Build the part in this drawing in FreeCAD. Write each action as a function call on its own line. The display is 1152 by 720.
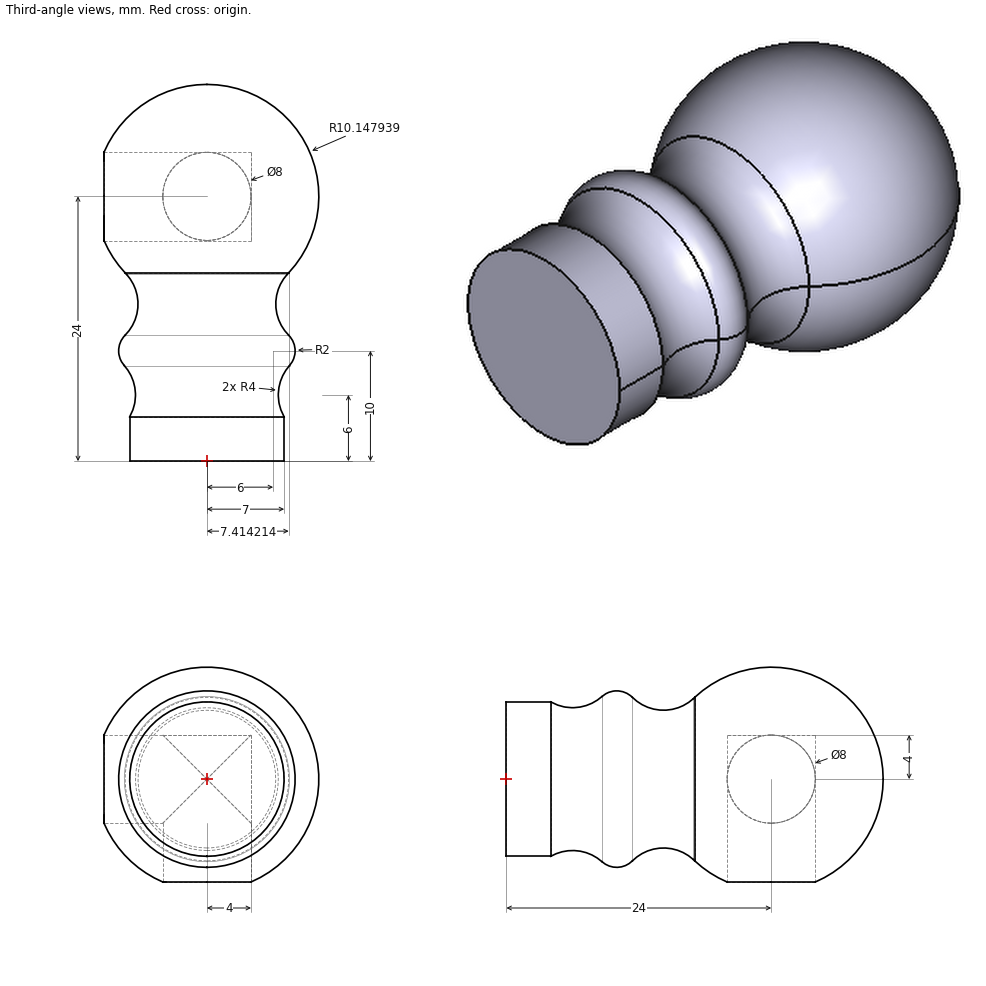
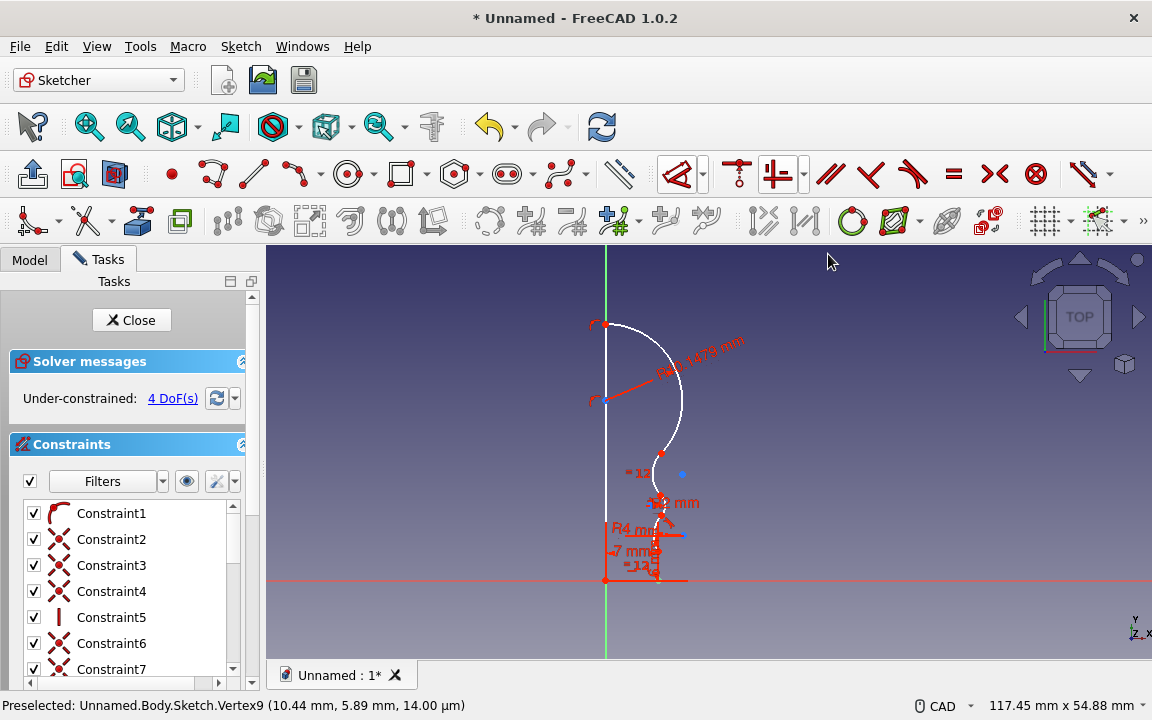
click(650, 506)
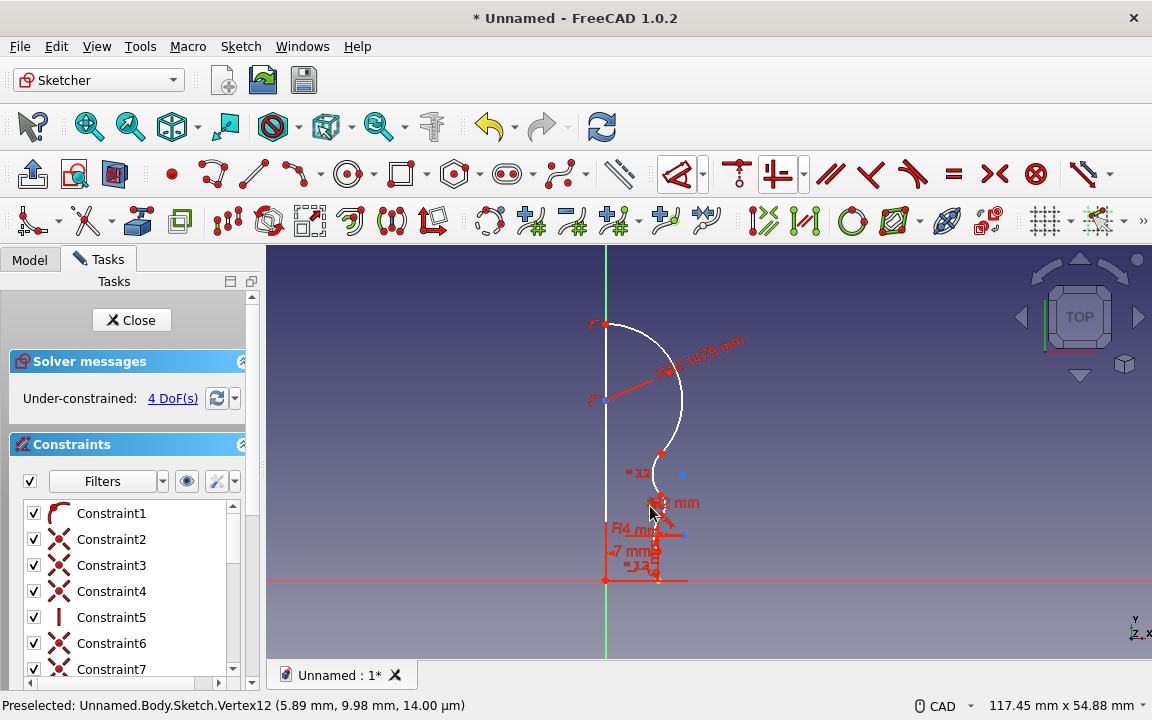
key(l)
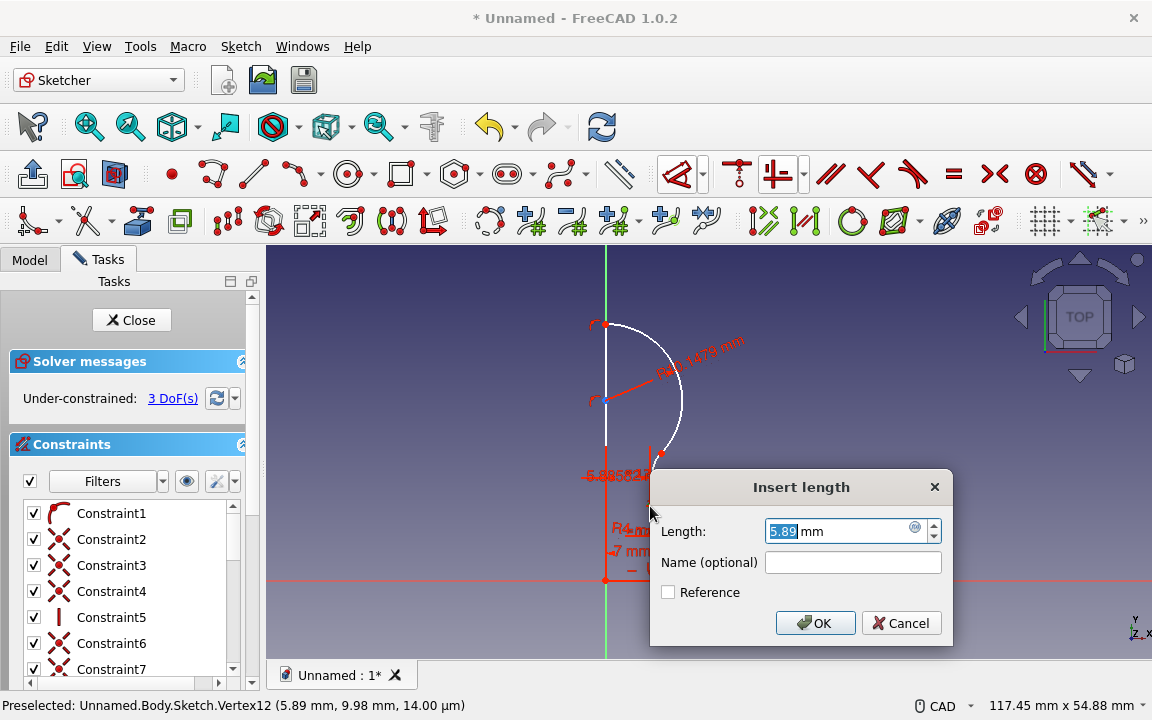
text(6)
key(Return)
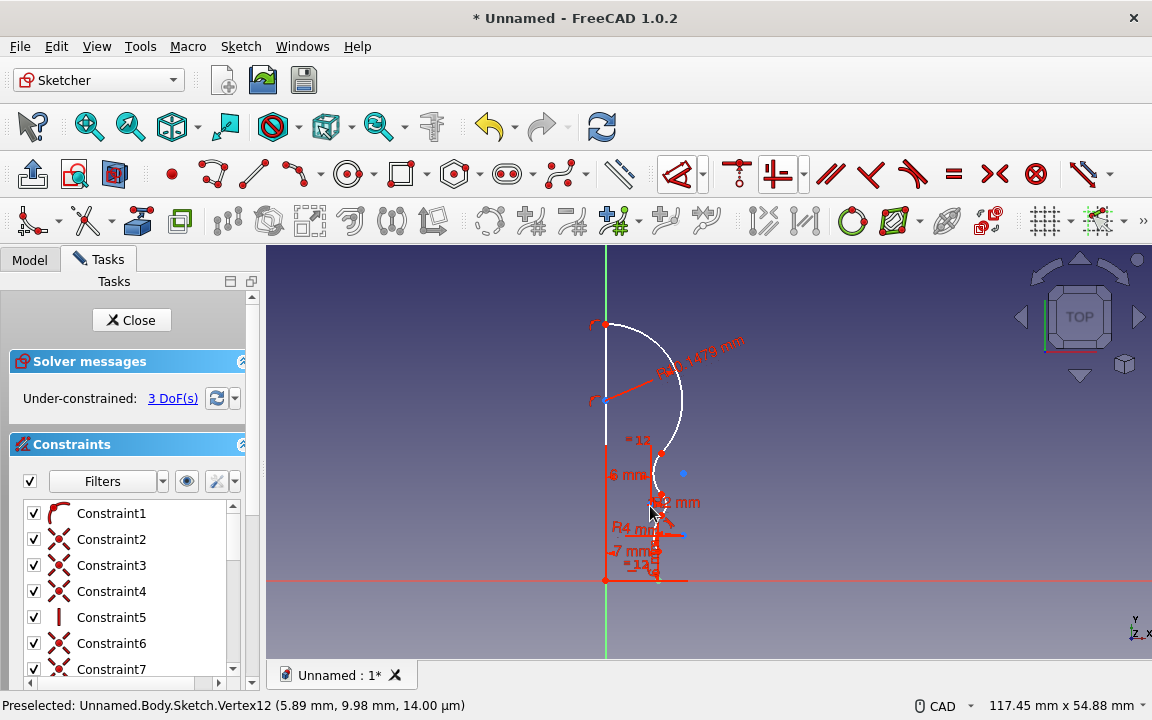
click(651, 505)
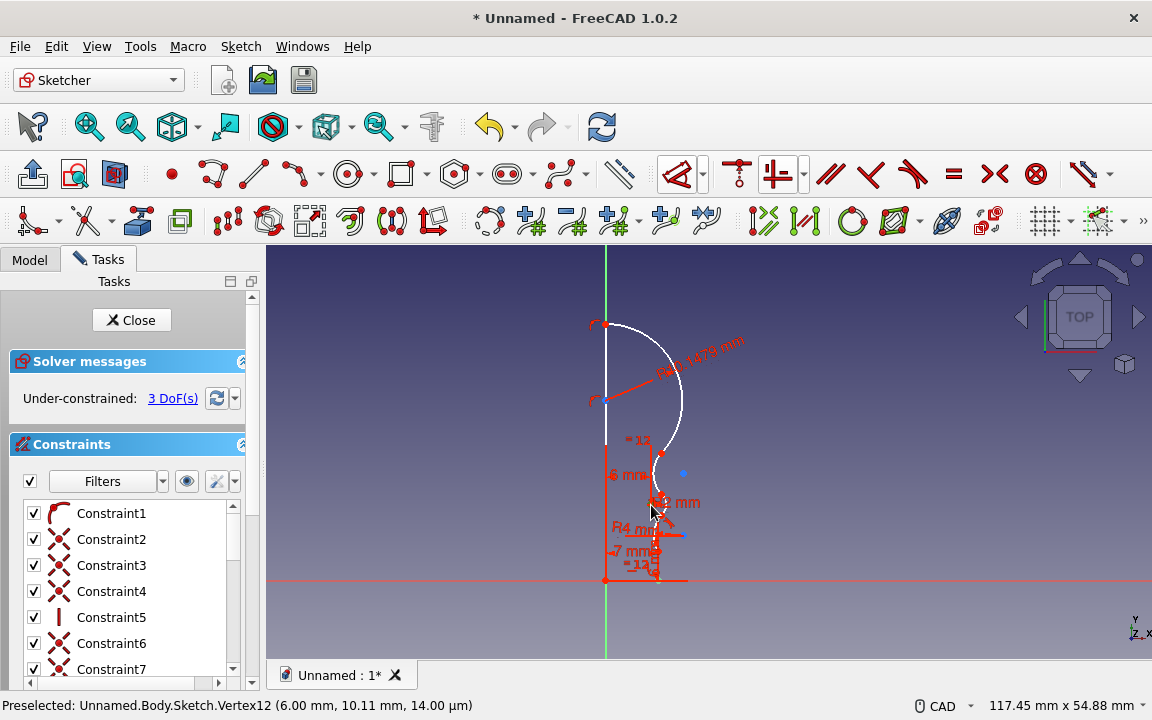
key(i)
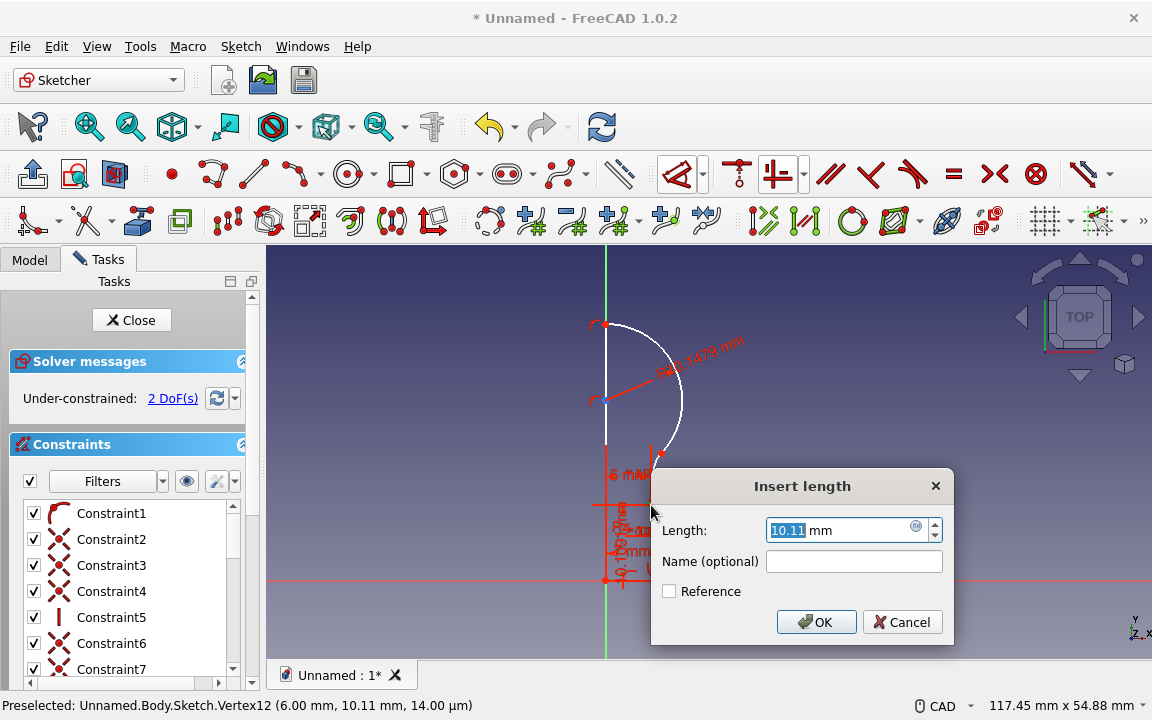
text(10)
key(Return)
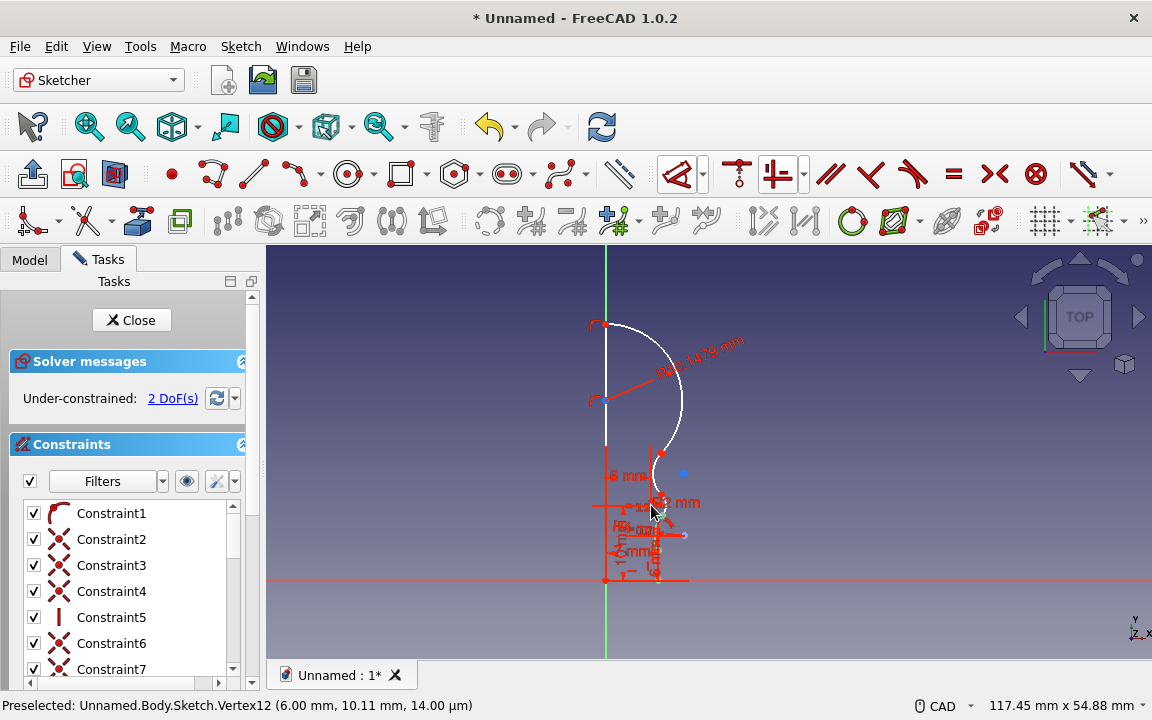
click(606, 401)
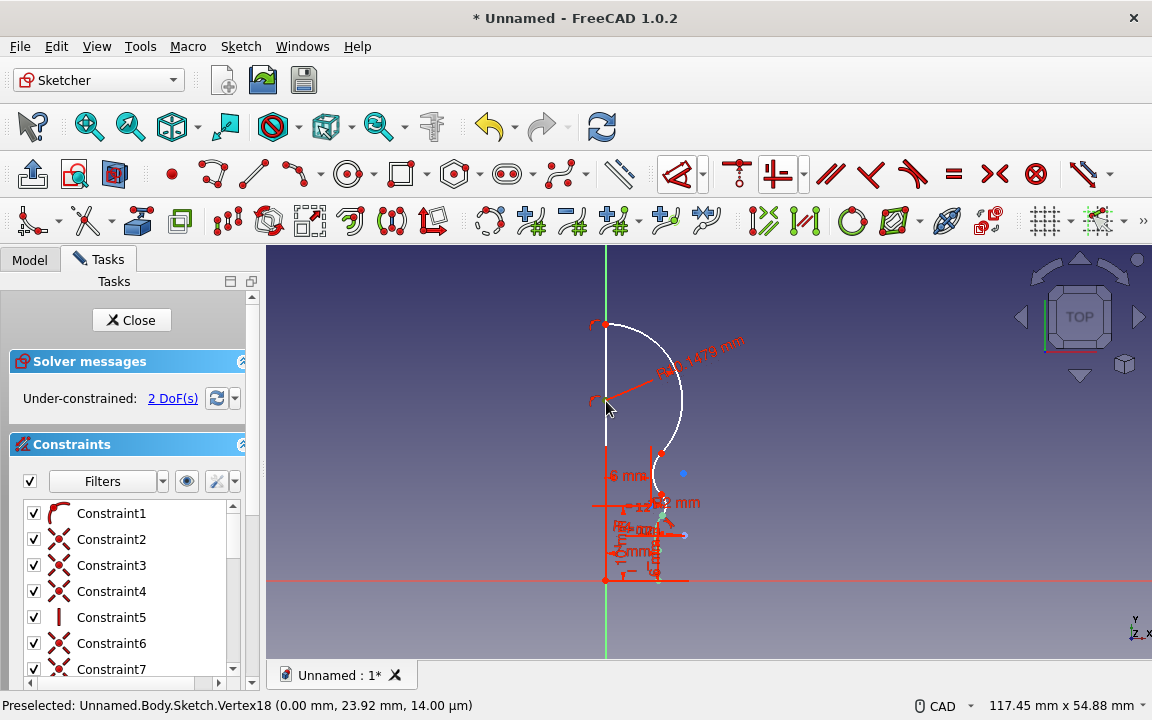
key(i)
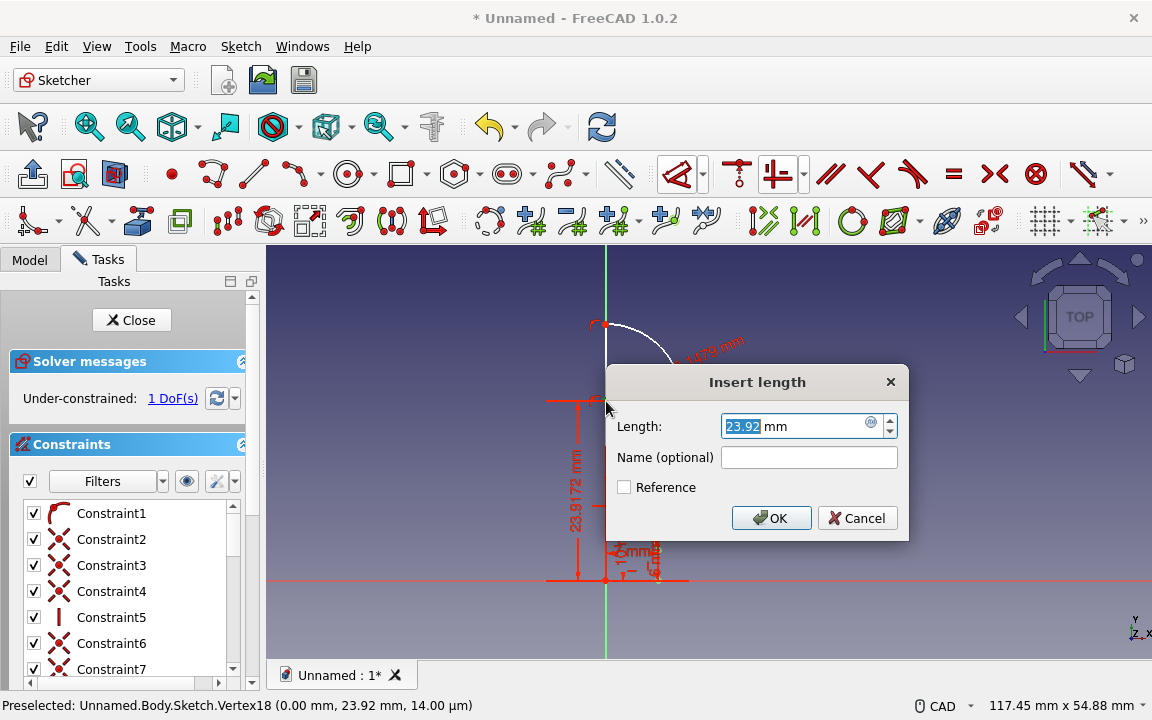
text(24)
key(Return)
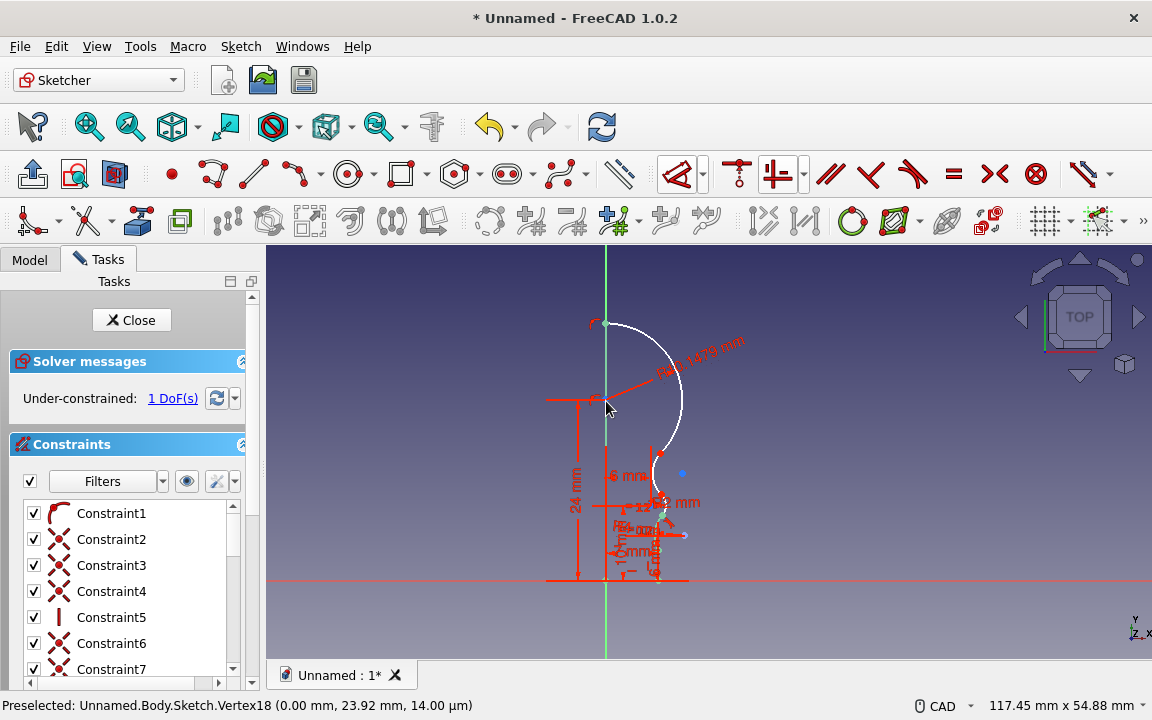
click(661, 453)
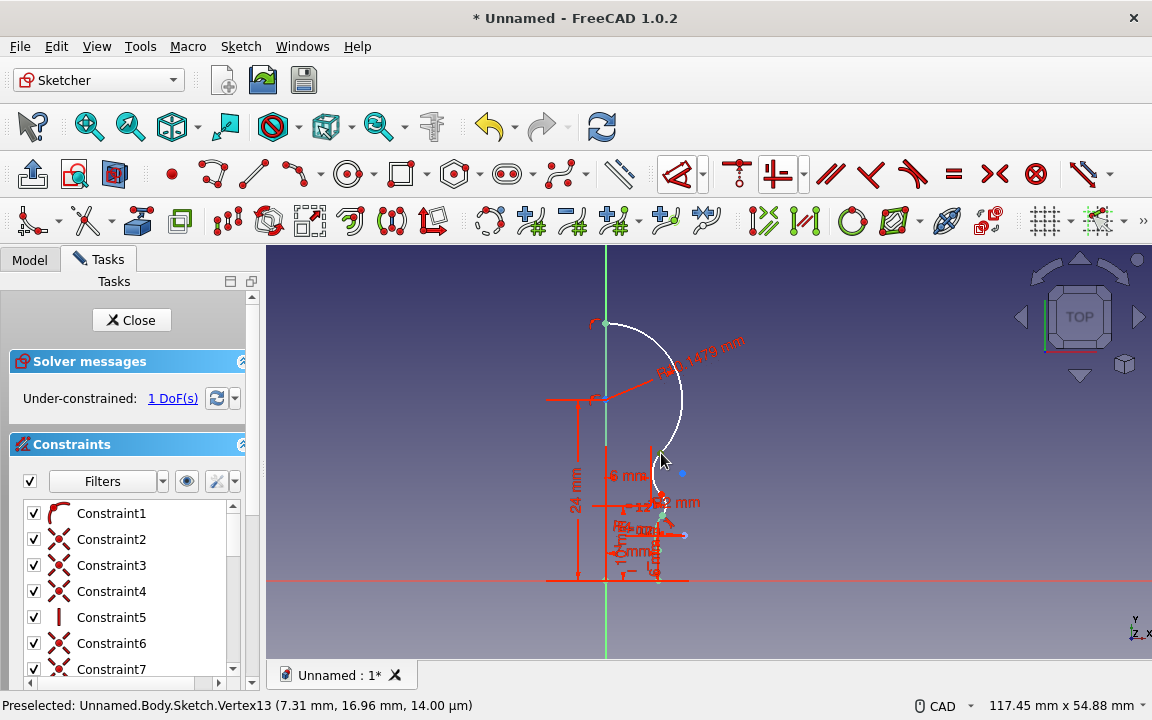
click(702, 174)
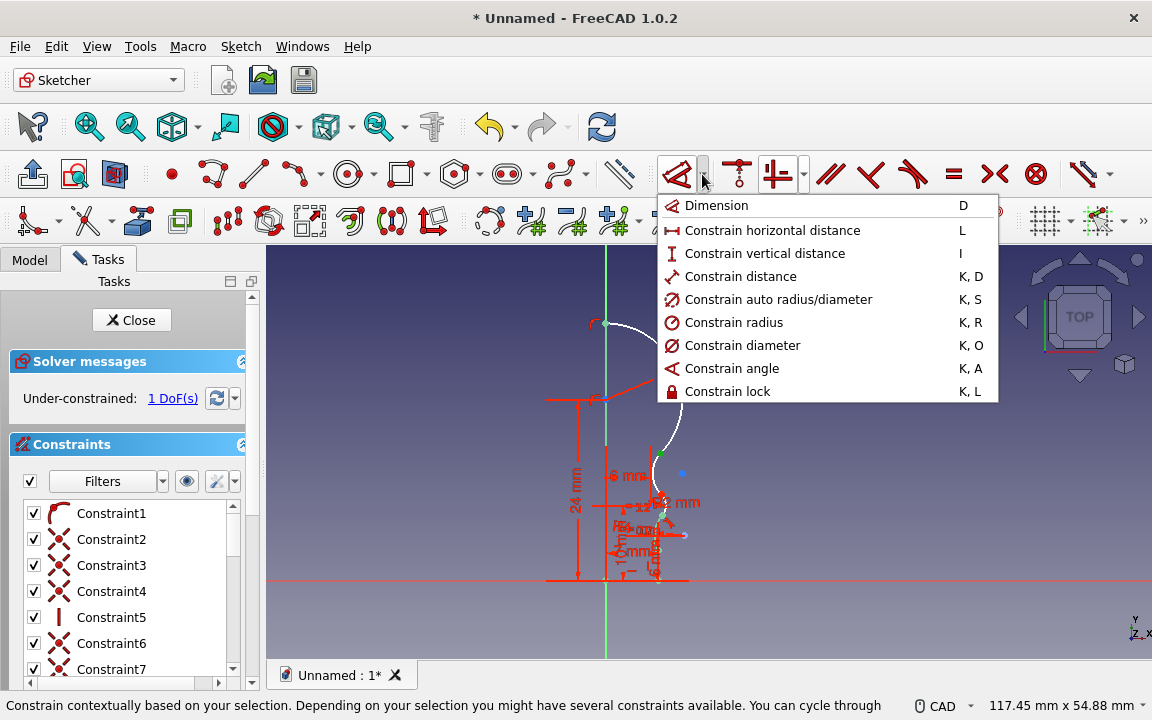
click(828, 230)